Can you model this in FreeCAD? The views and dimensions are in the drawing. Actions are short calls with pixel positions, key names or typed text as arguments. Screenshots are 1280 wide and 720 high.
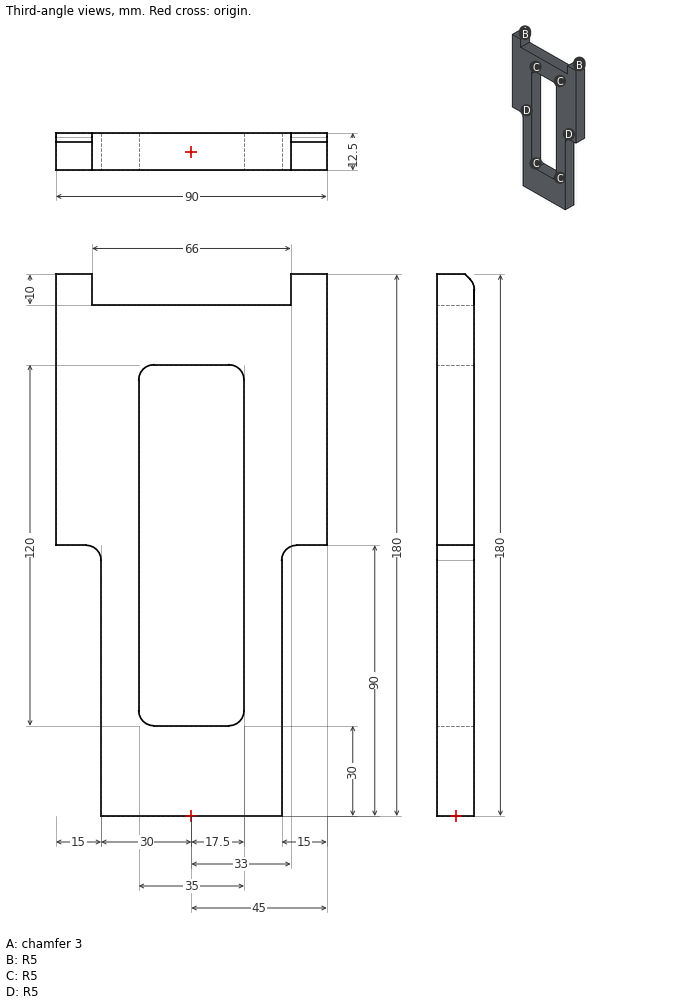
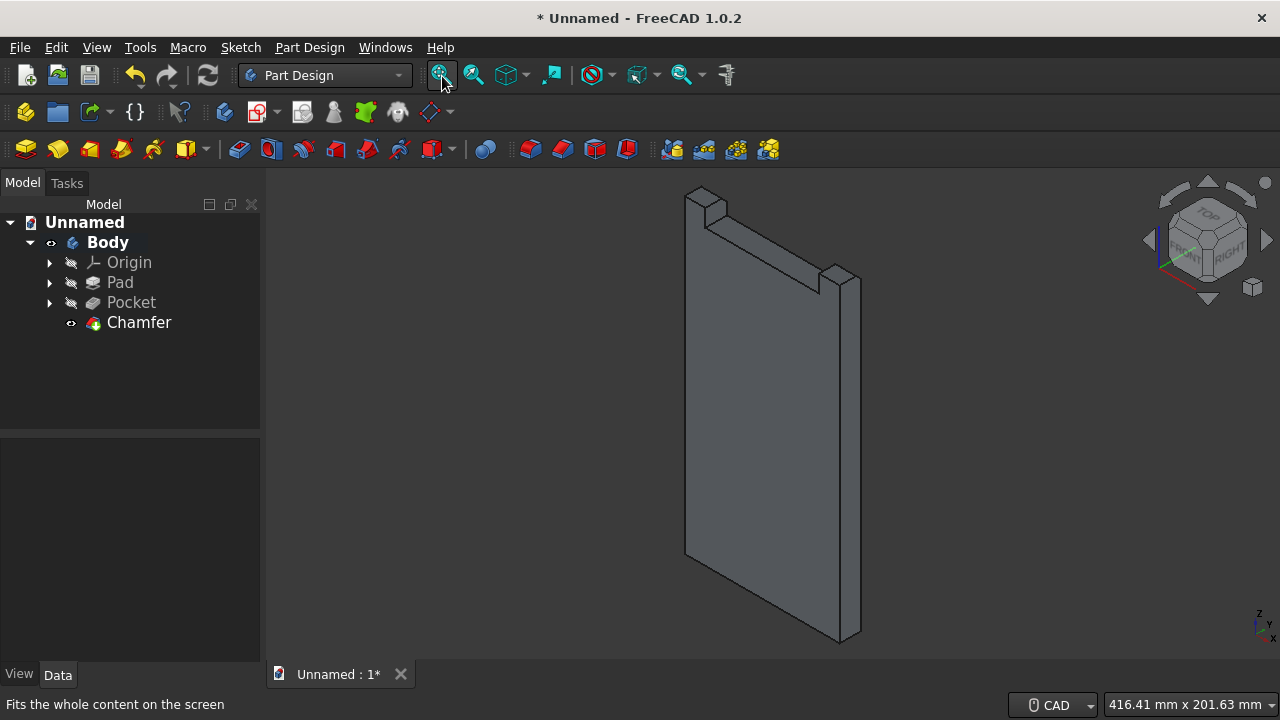
key(2)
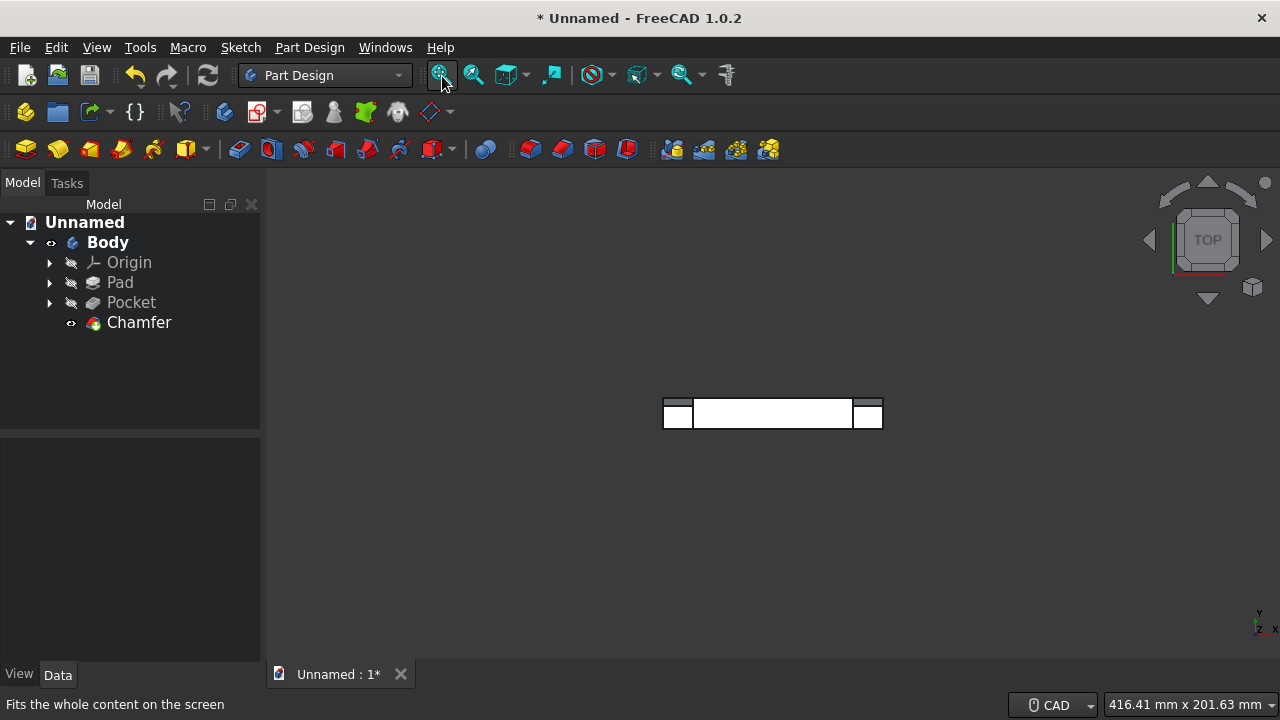
click(442, 76)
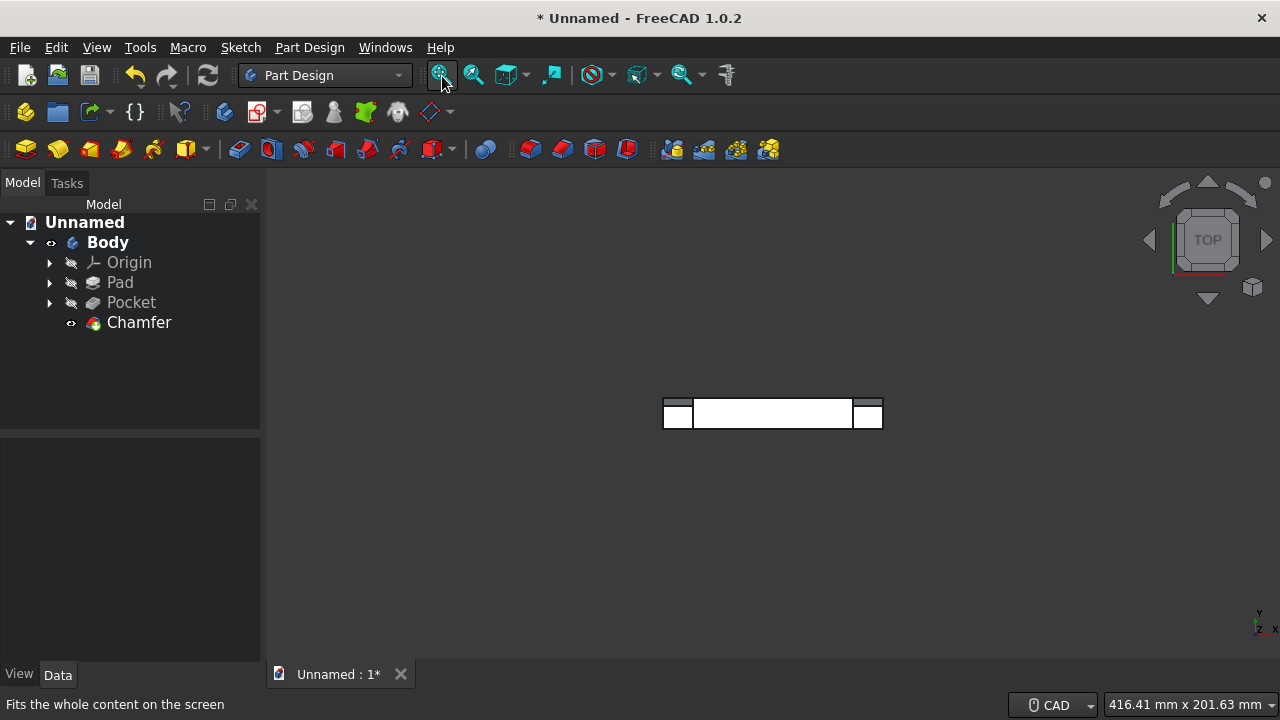
key(1)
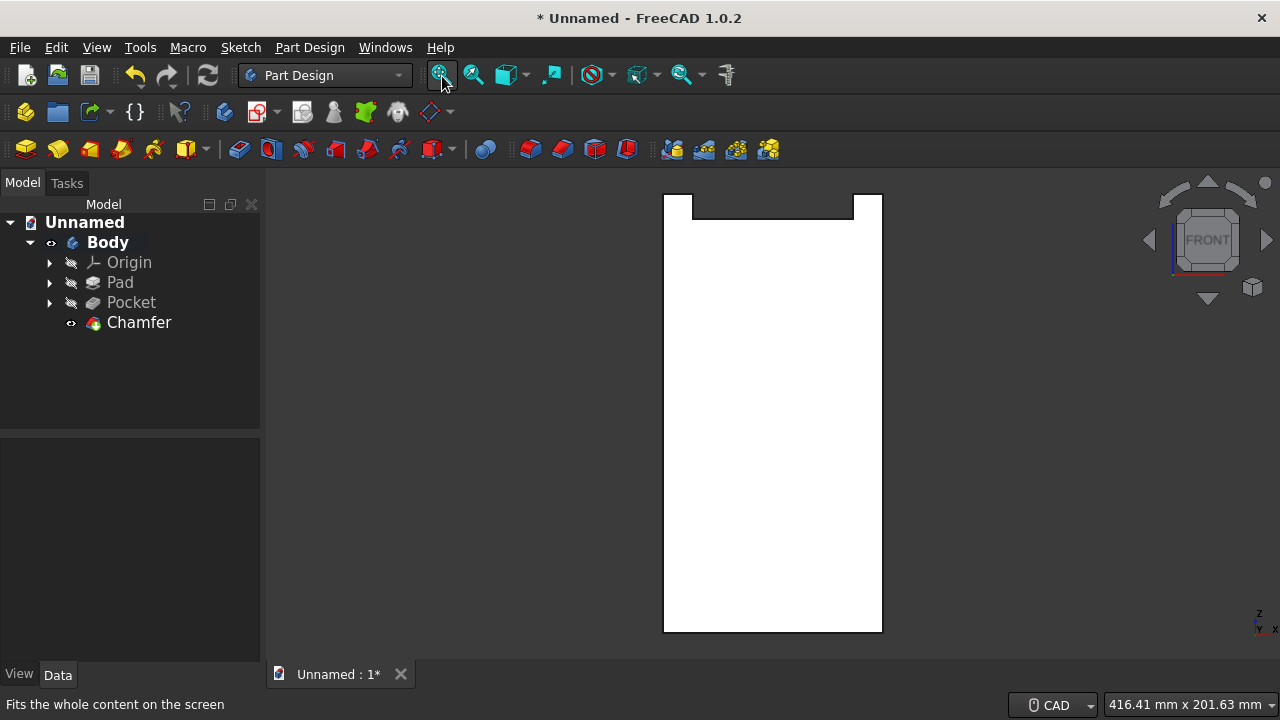
key(3)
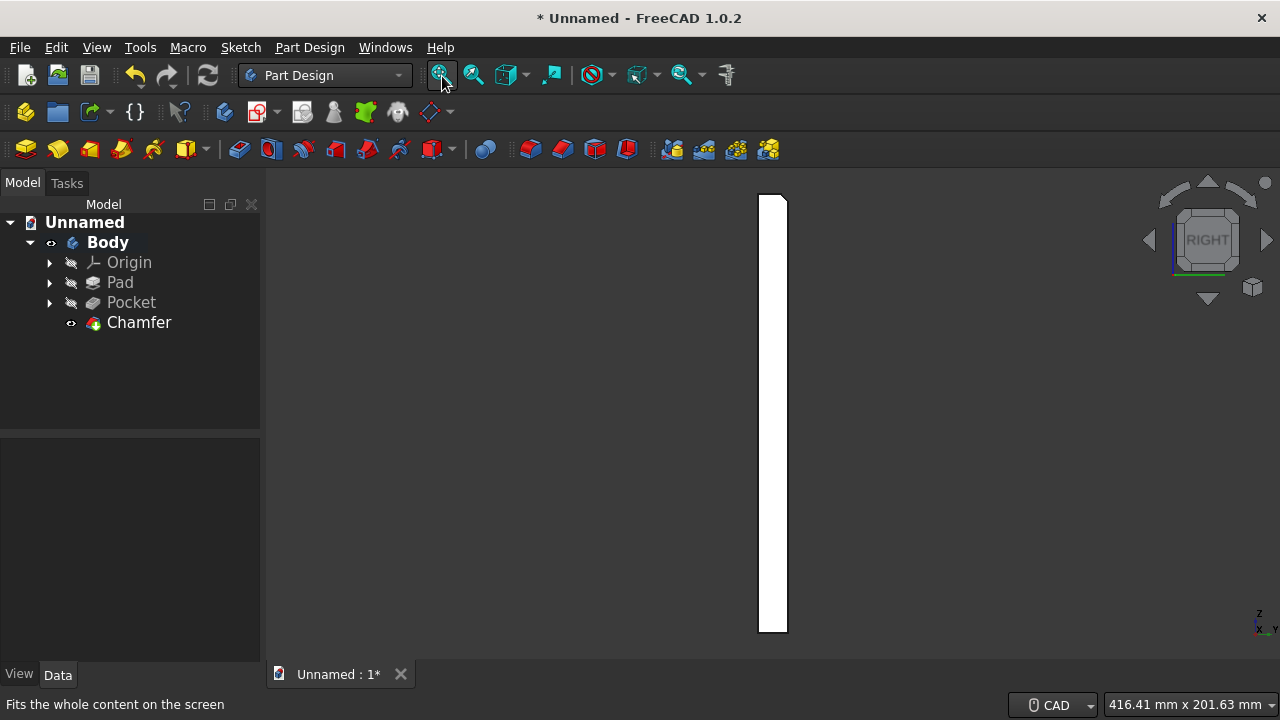
key(5)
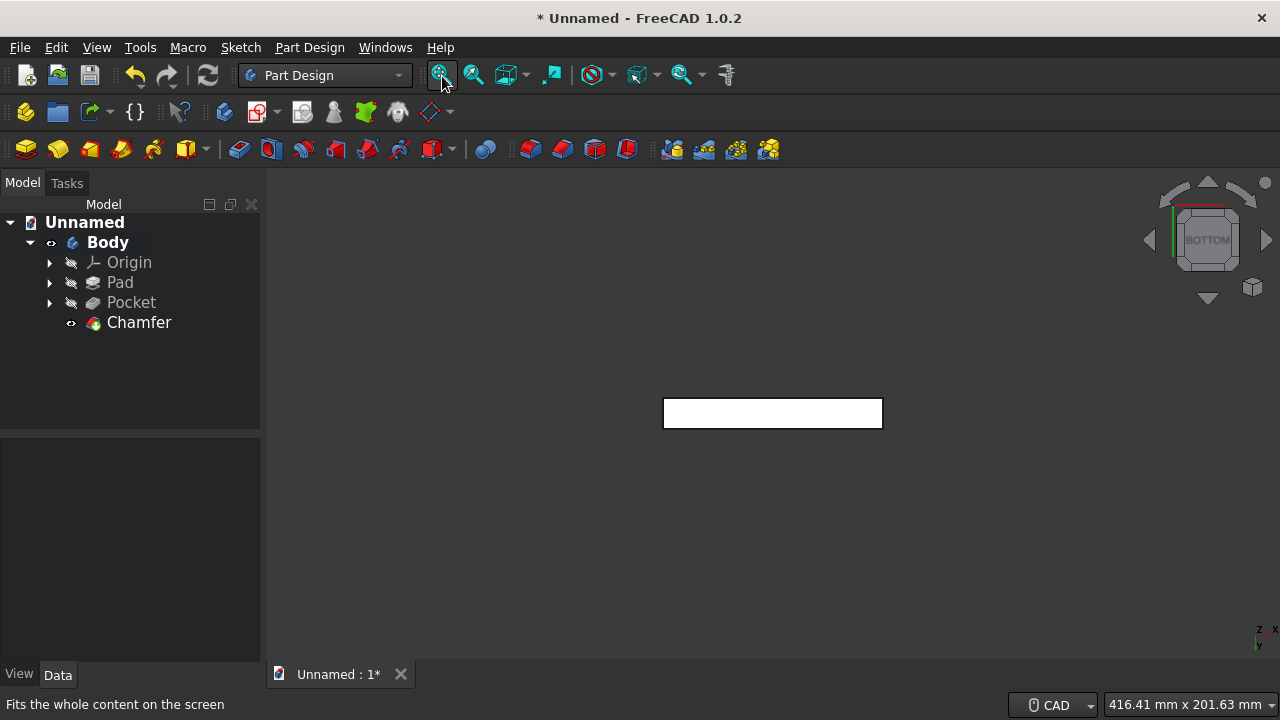
click(442, 76)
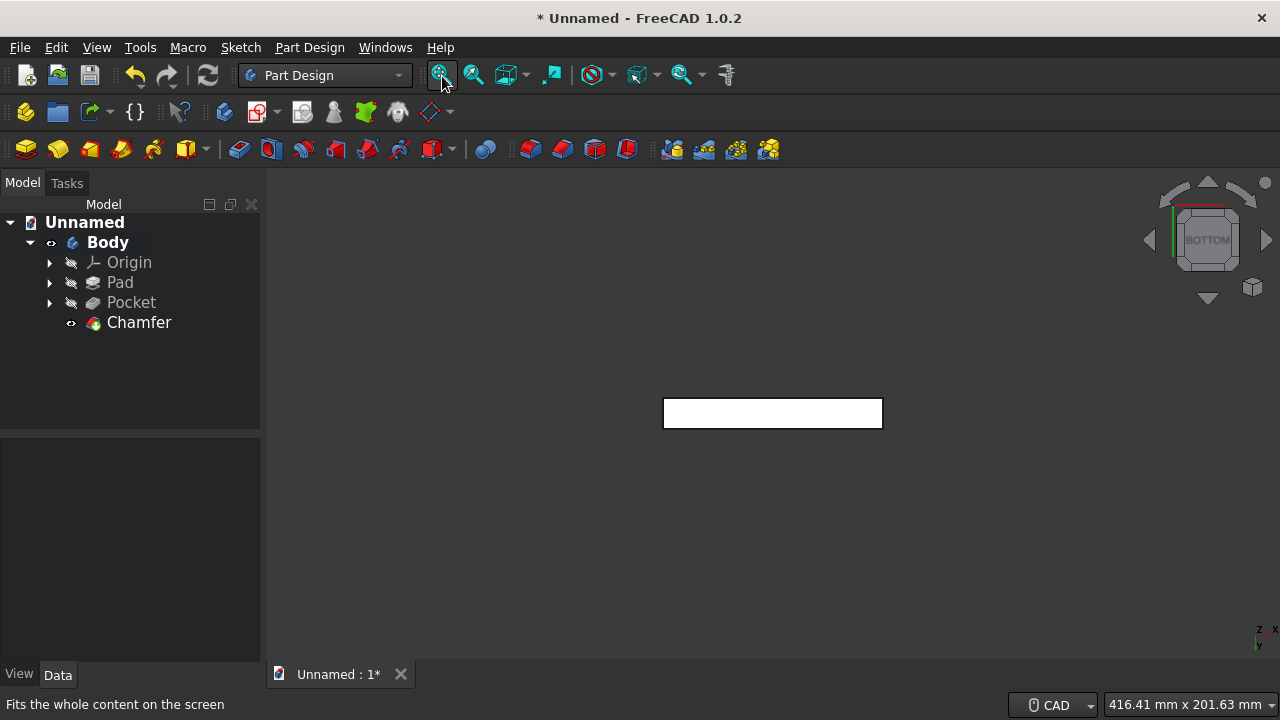
key(4)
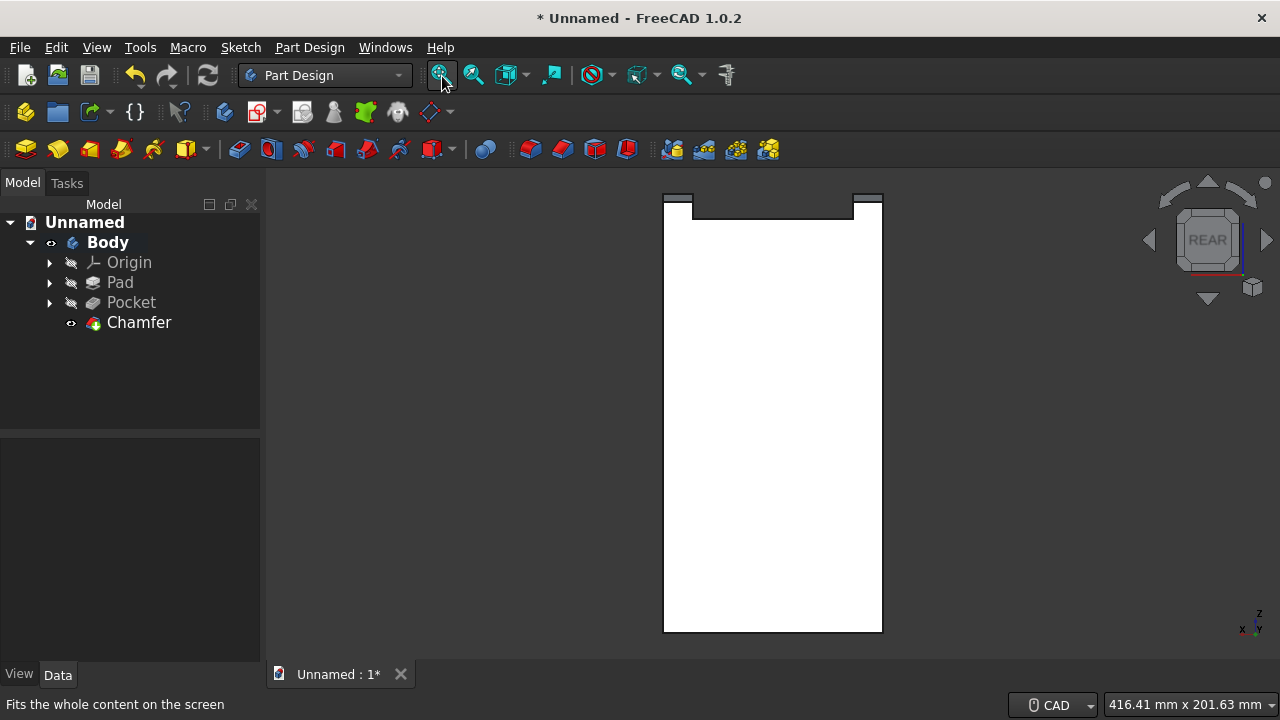
click(678, 201)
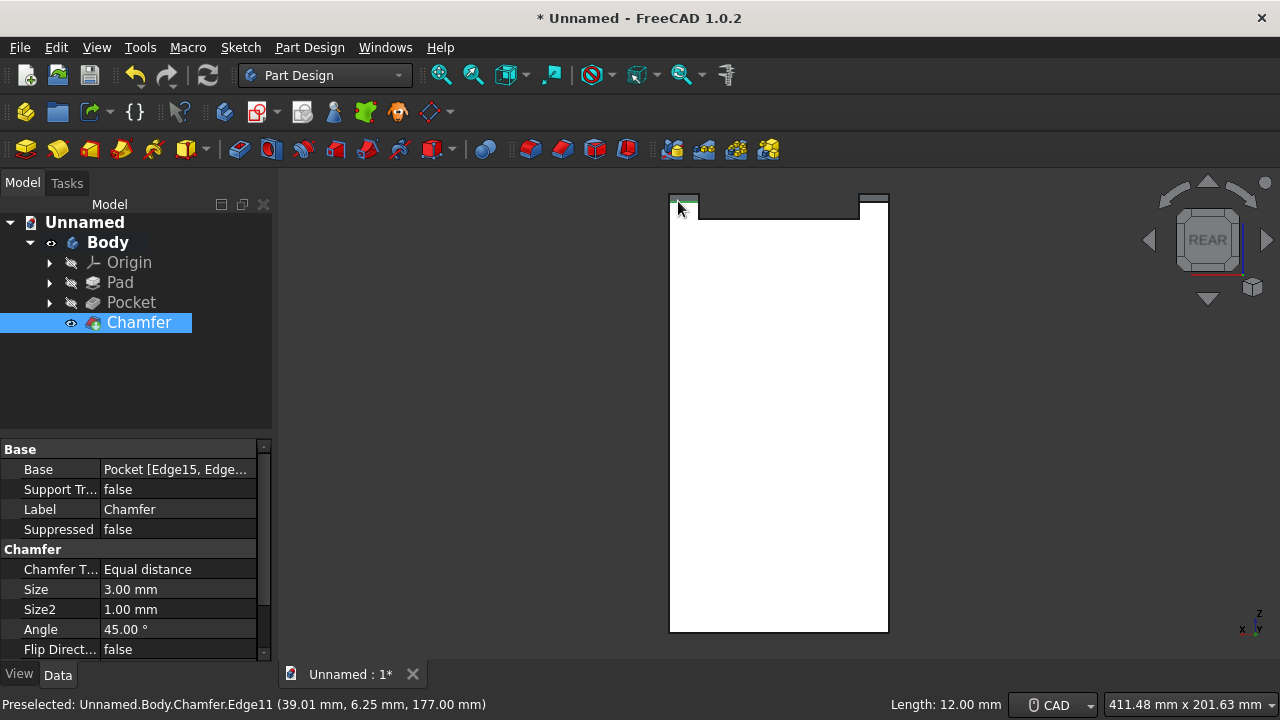
click(874, 201, ctrl)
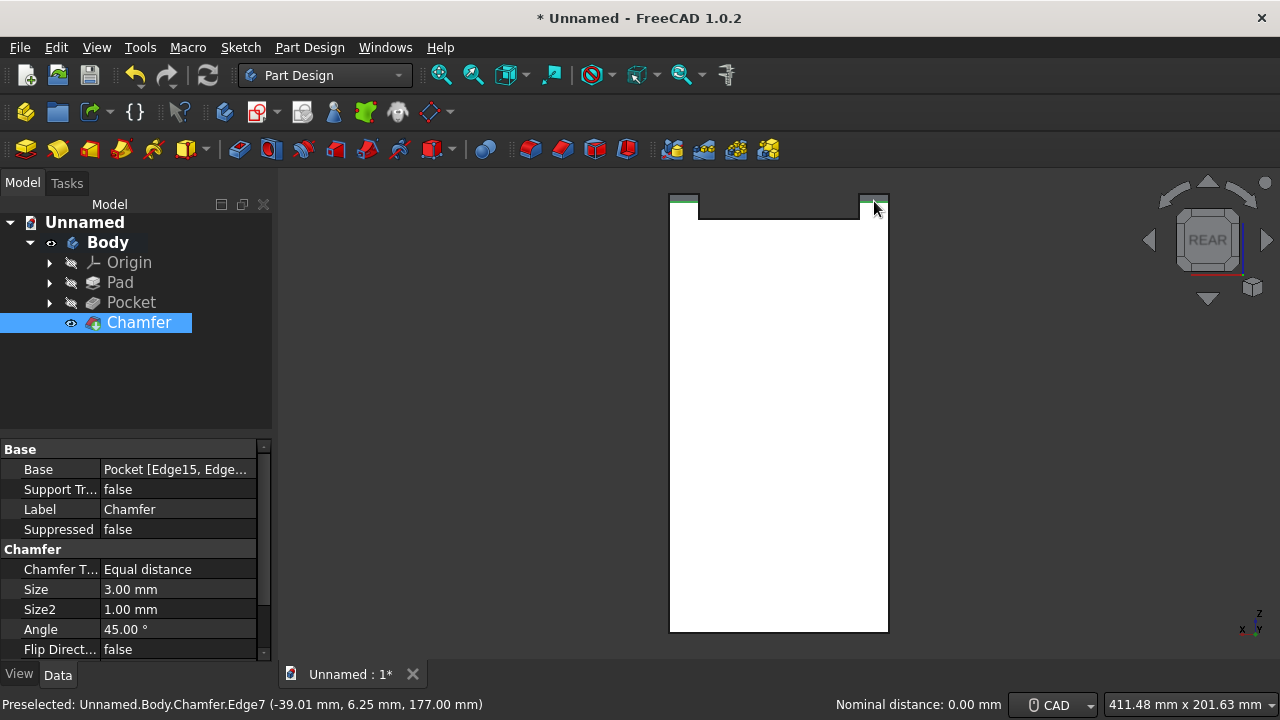
click(532, 150)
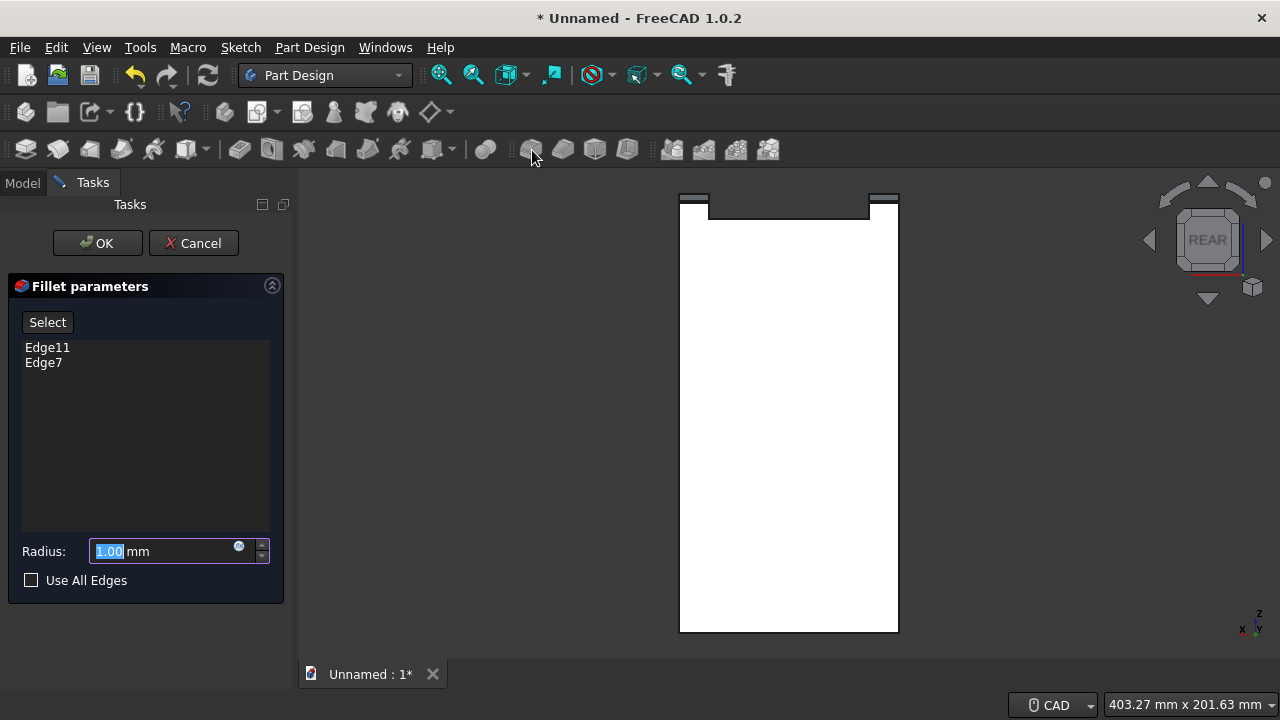
text(5)
key(Tab)